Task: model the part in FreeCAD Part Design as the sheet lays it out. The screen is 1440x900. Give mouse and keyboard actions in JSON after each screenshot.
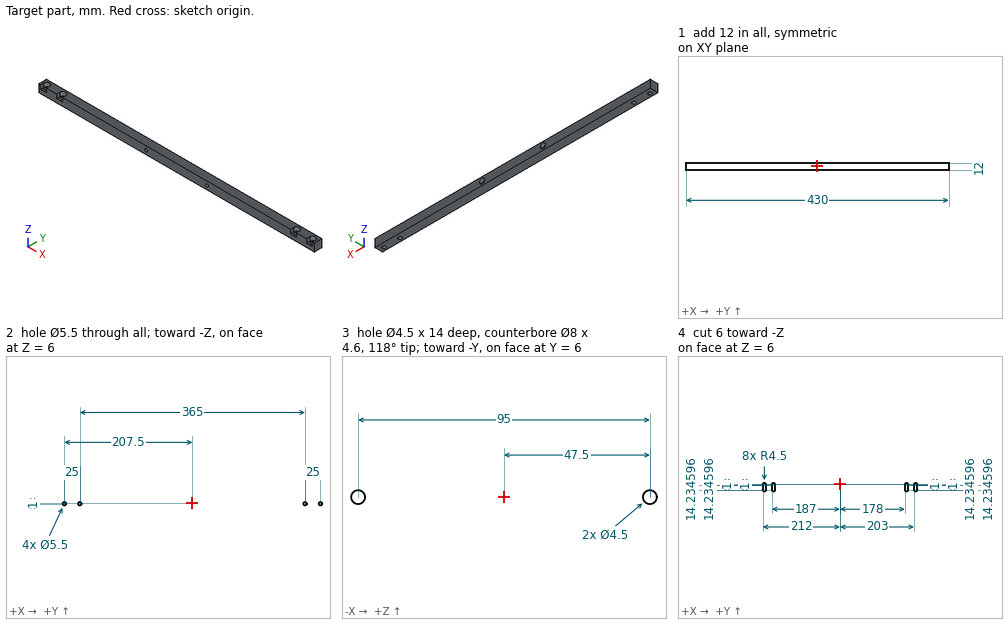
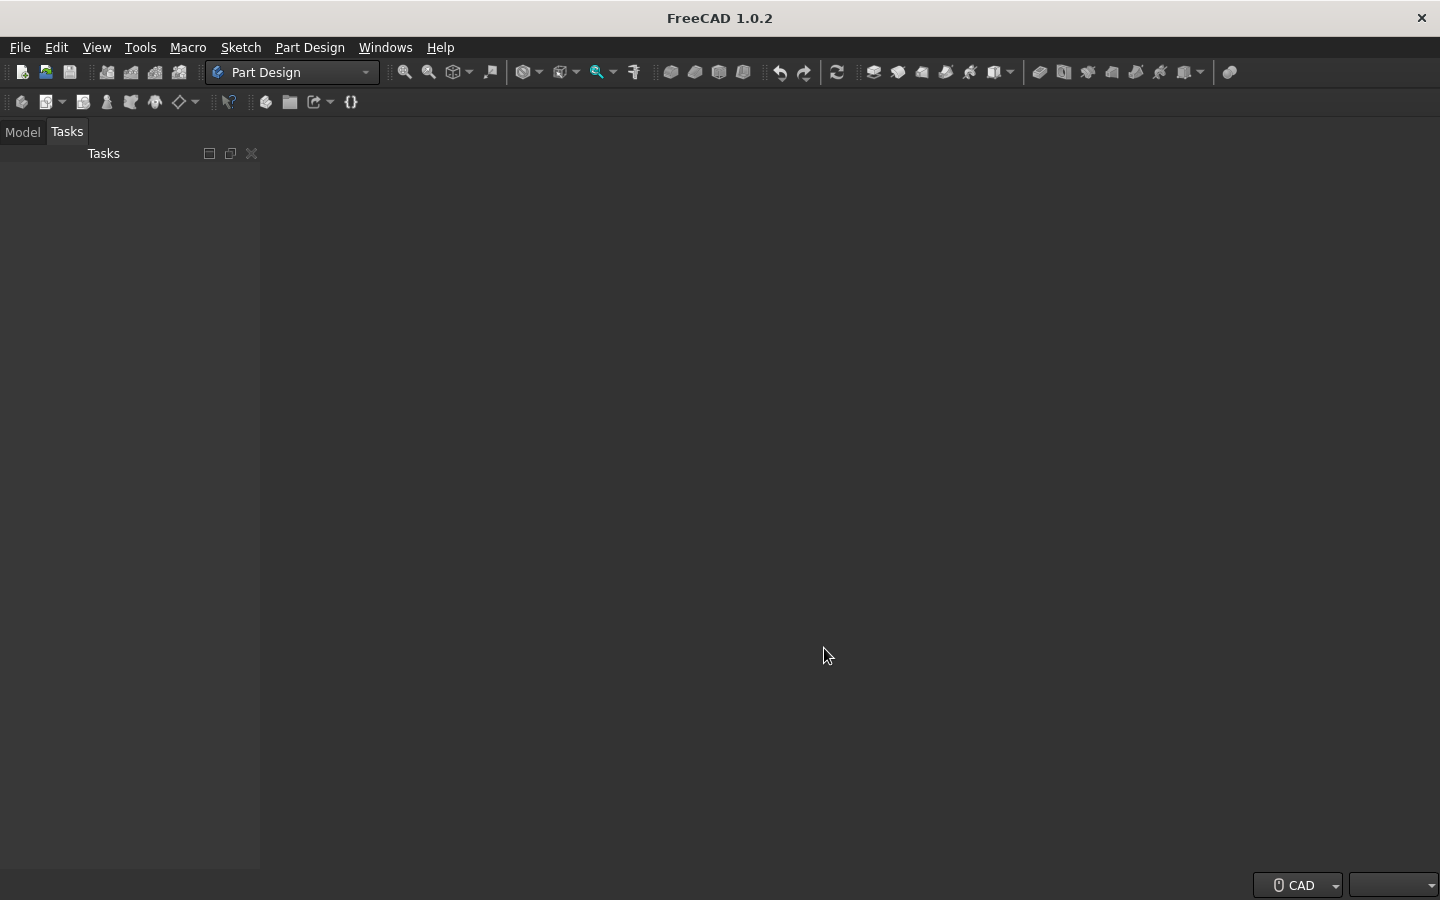
{"action": "left_click", "coordinate": [22, 72]}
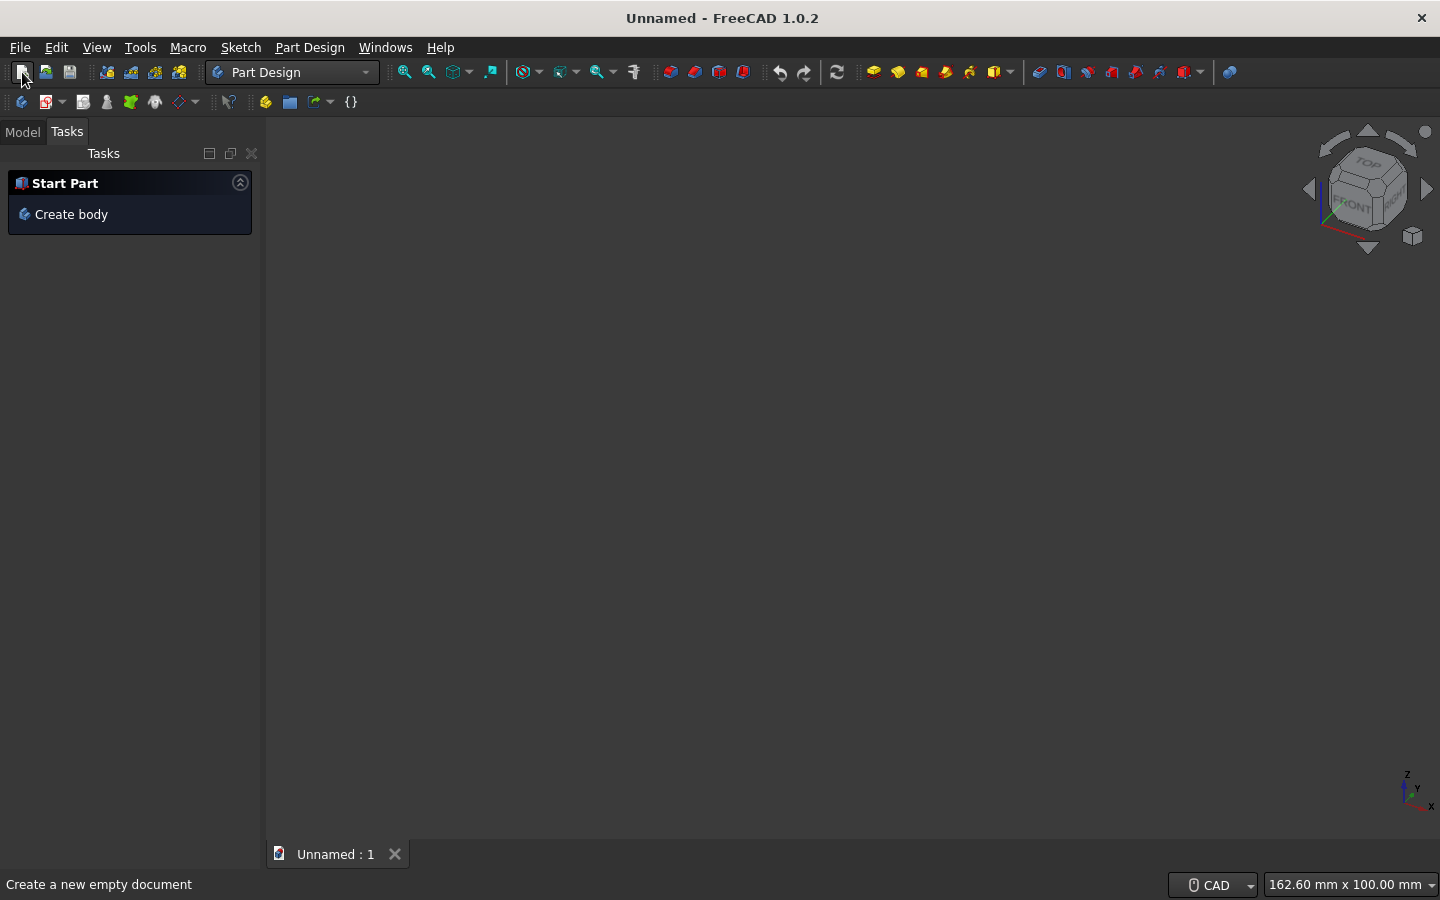
{"action": "left_click", "coordinate": [46, 102]}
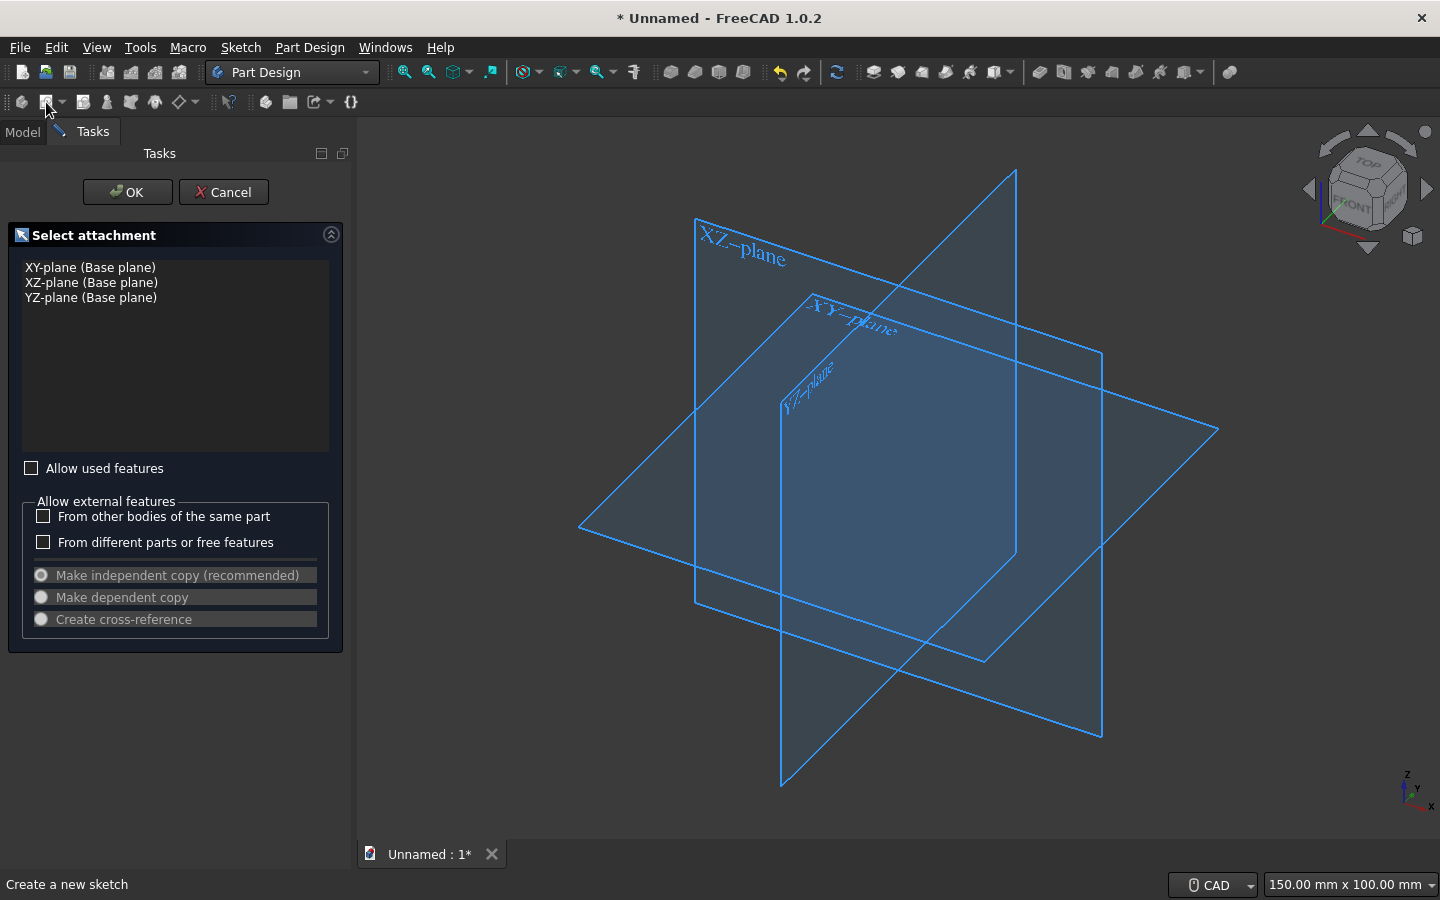
{"action": "left_click", "coordinate": [82, 268]}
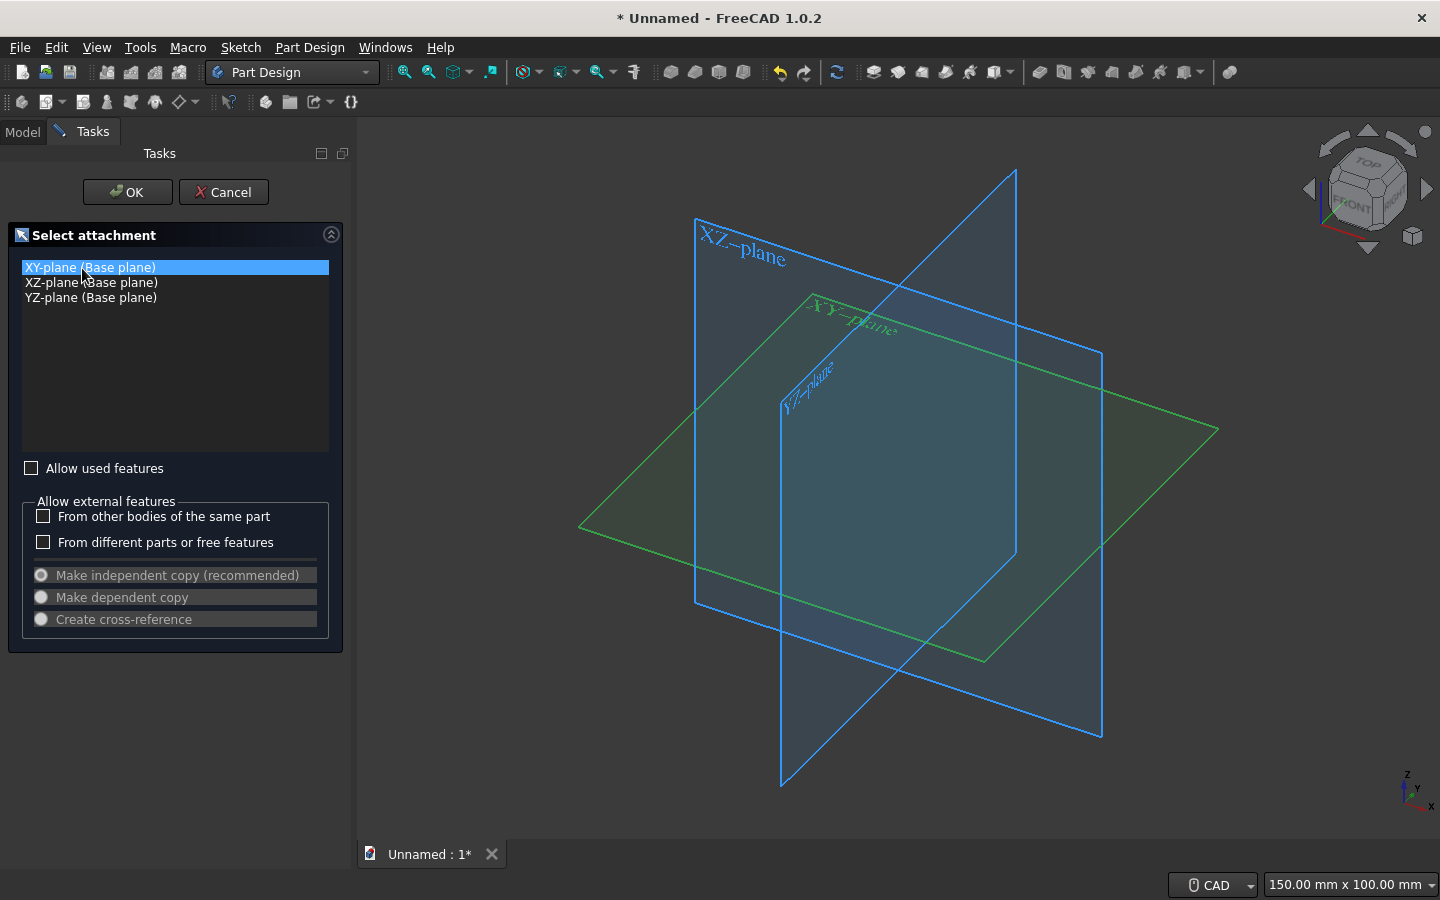
{"action": "left_click", "coordinate": [128, 192]}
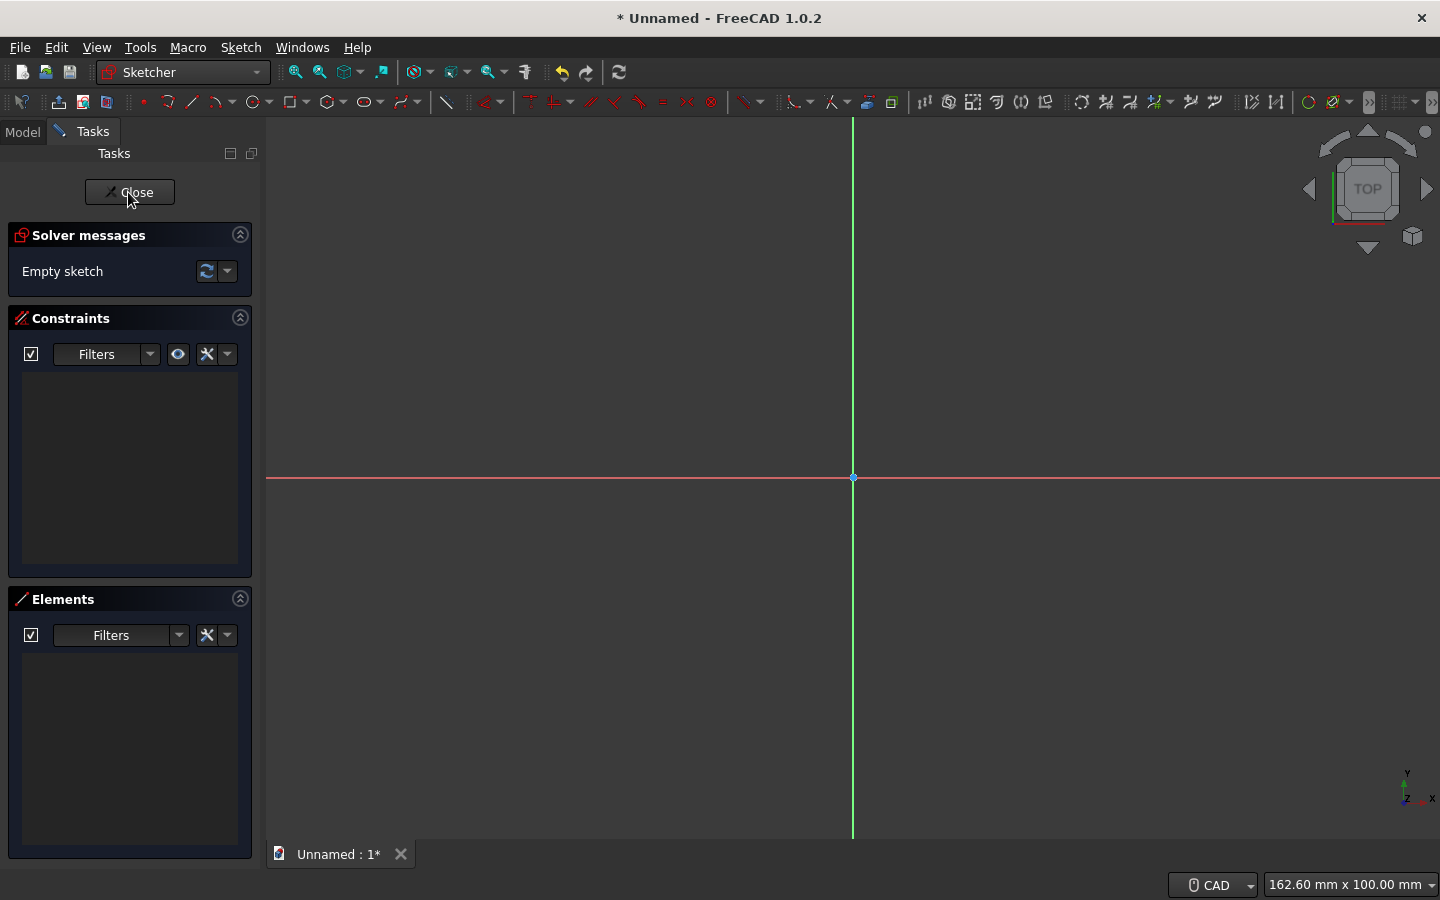
{"action": "scroll", "coordinate": [767, 478], "scroll_direction": "down", "scroll_amount": 8}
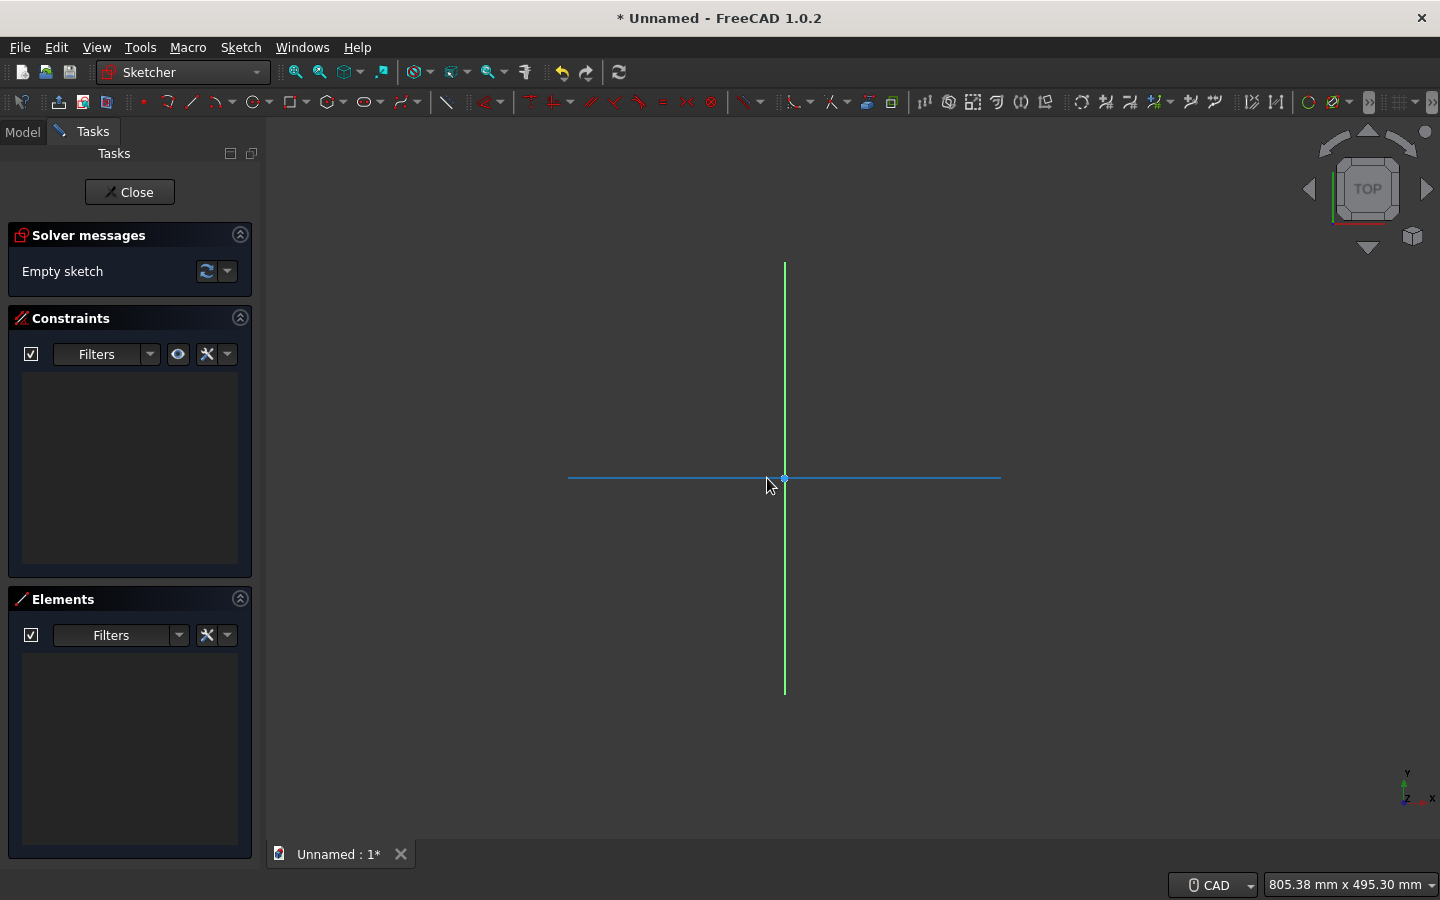
{"action": "left_click", "coordinate": [308, 102]}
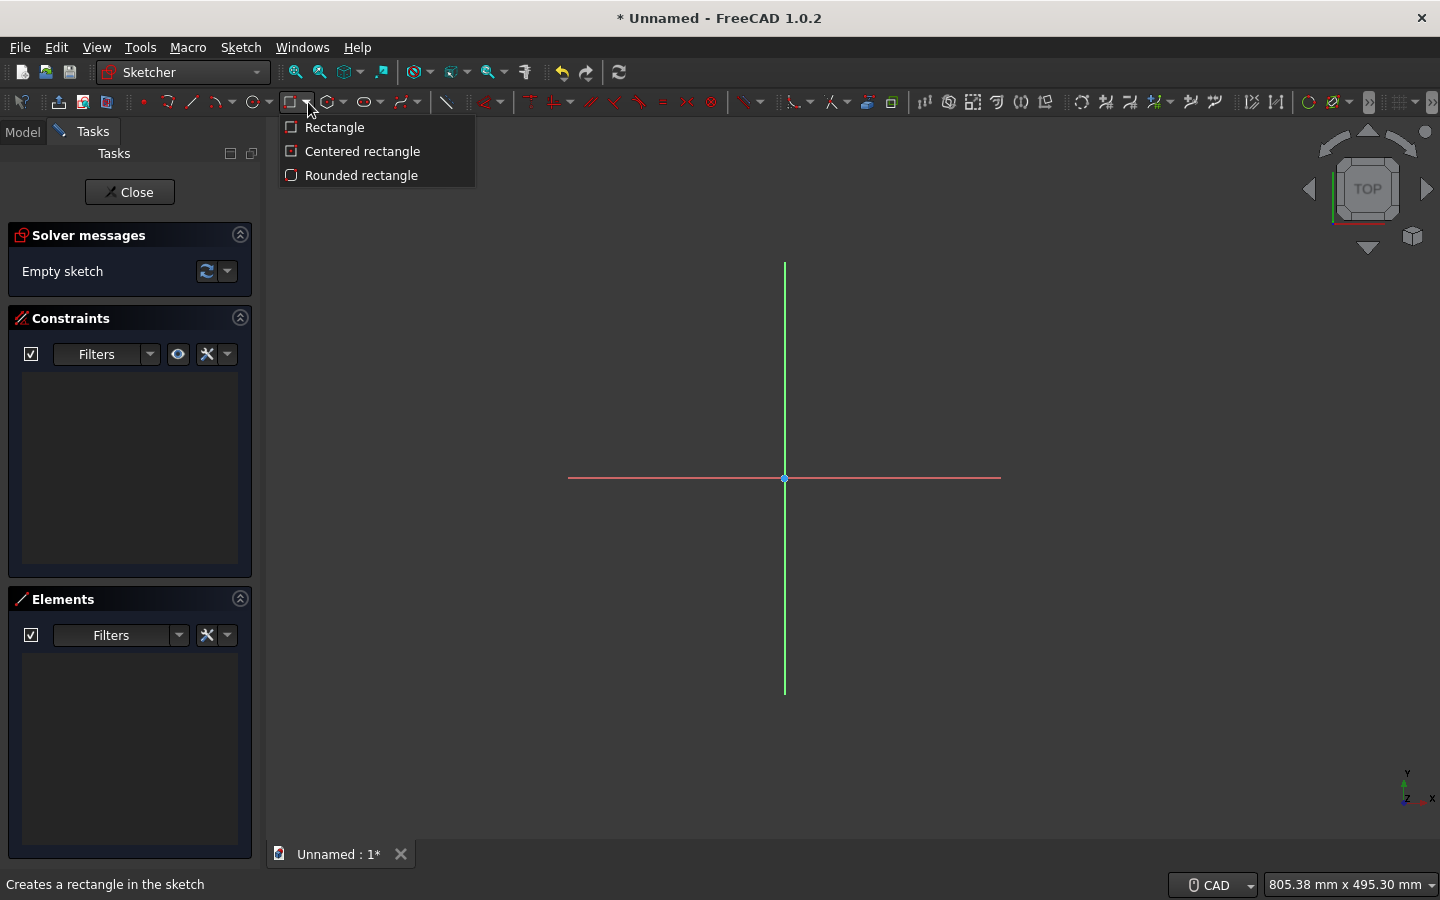
{"action": "left_click", "coordinate": [378, 151]}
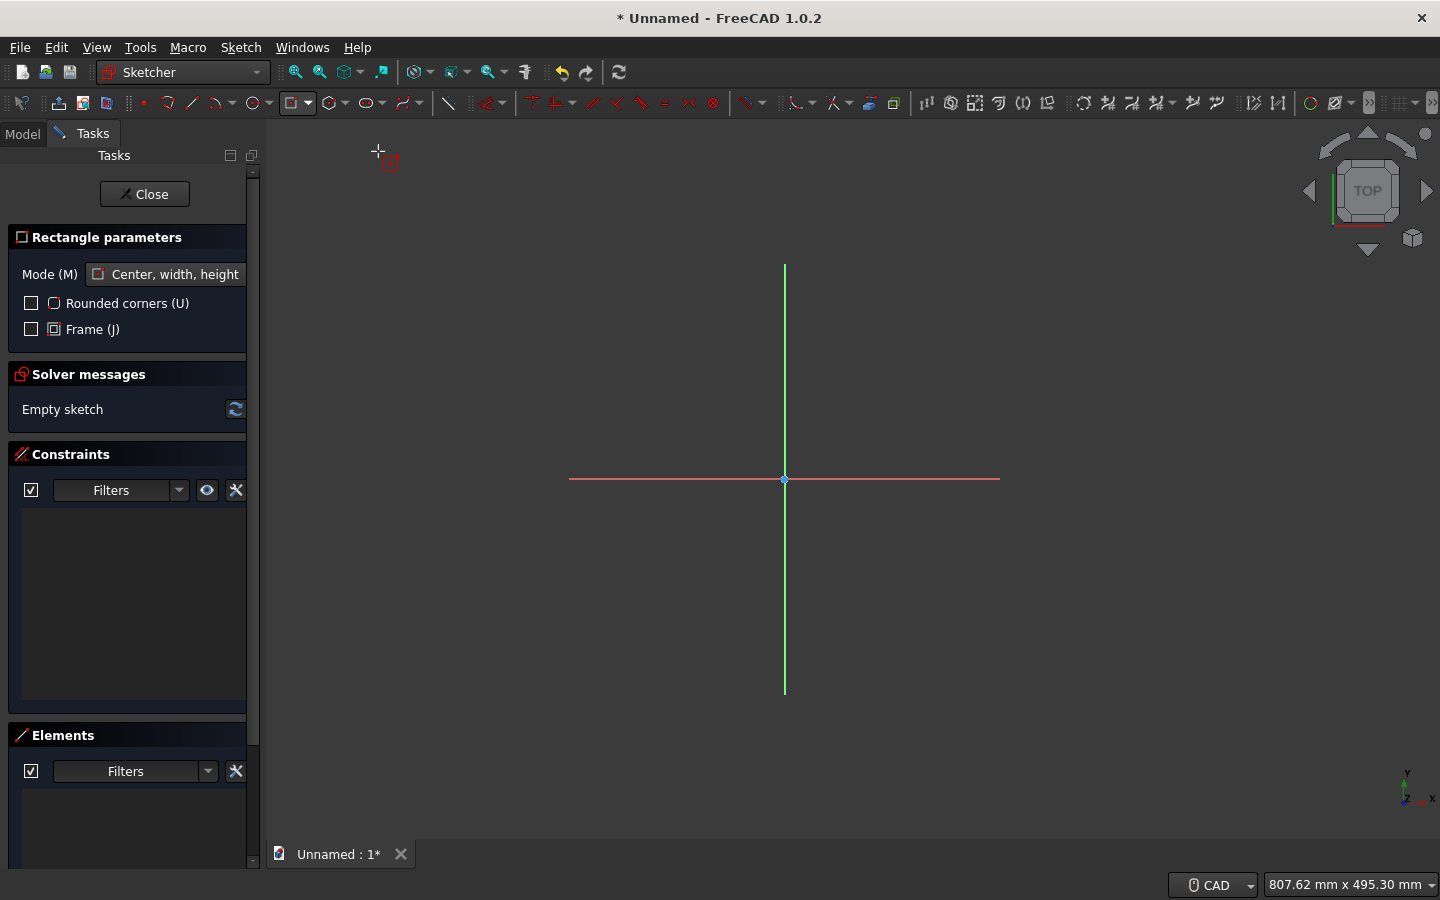
{"action": "scroll", "coordinate": [785, 479], "scroll_direction": "up", "scroll_amount": 3}